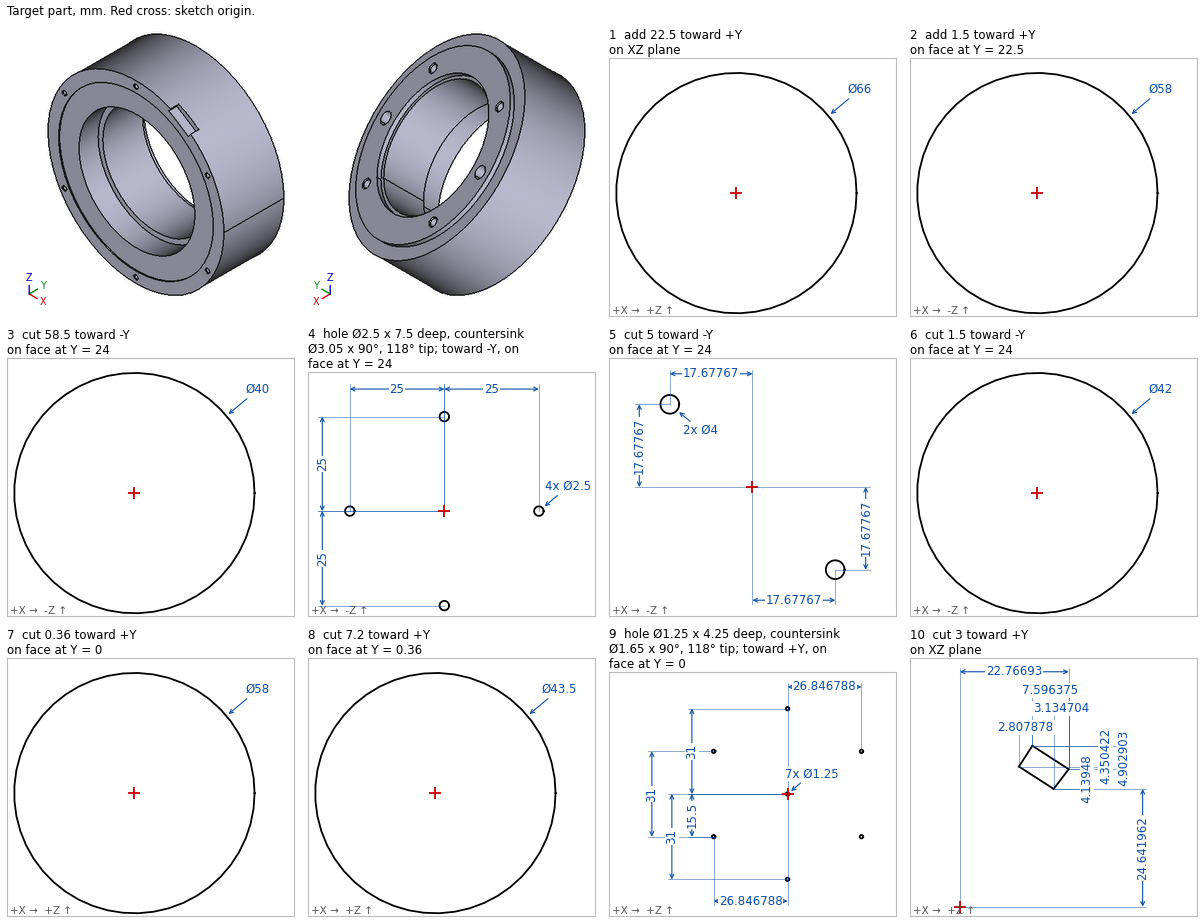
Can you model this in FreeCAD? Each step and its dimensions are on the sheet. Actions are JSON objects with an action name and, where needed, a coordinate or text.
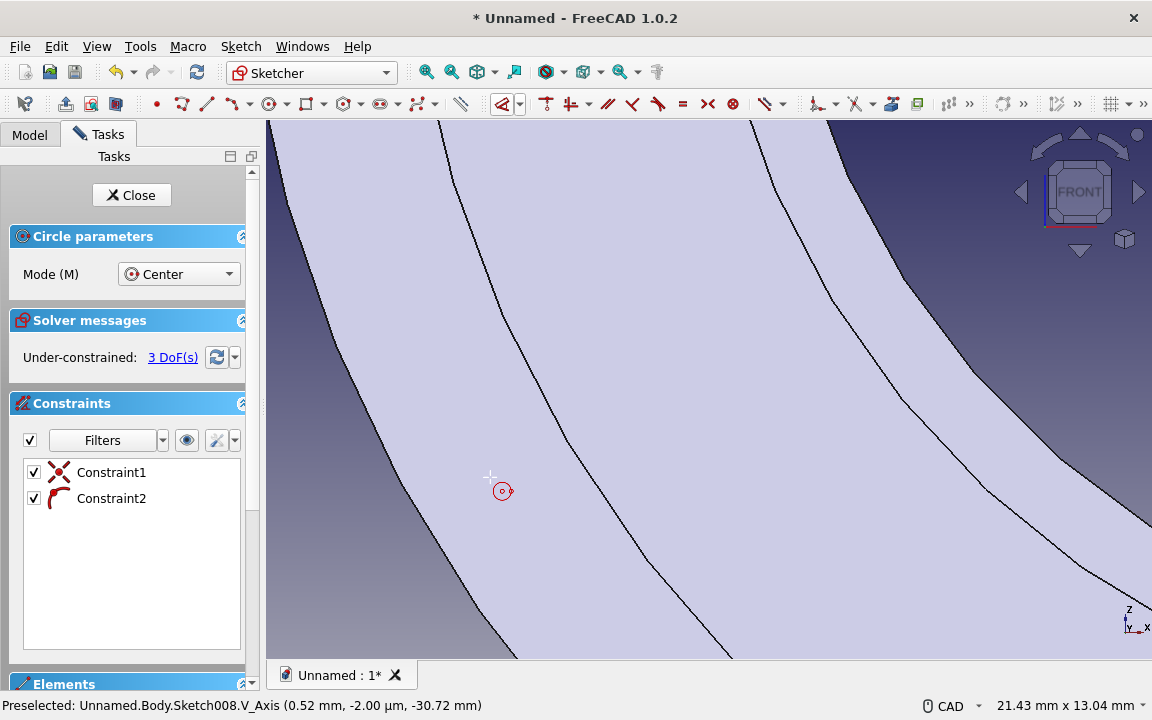
{"action": "scroll", "coordinate": [490, 477], "scroll_direction": "down", "scroll_amount": 10}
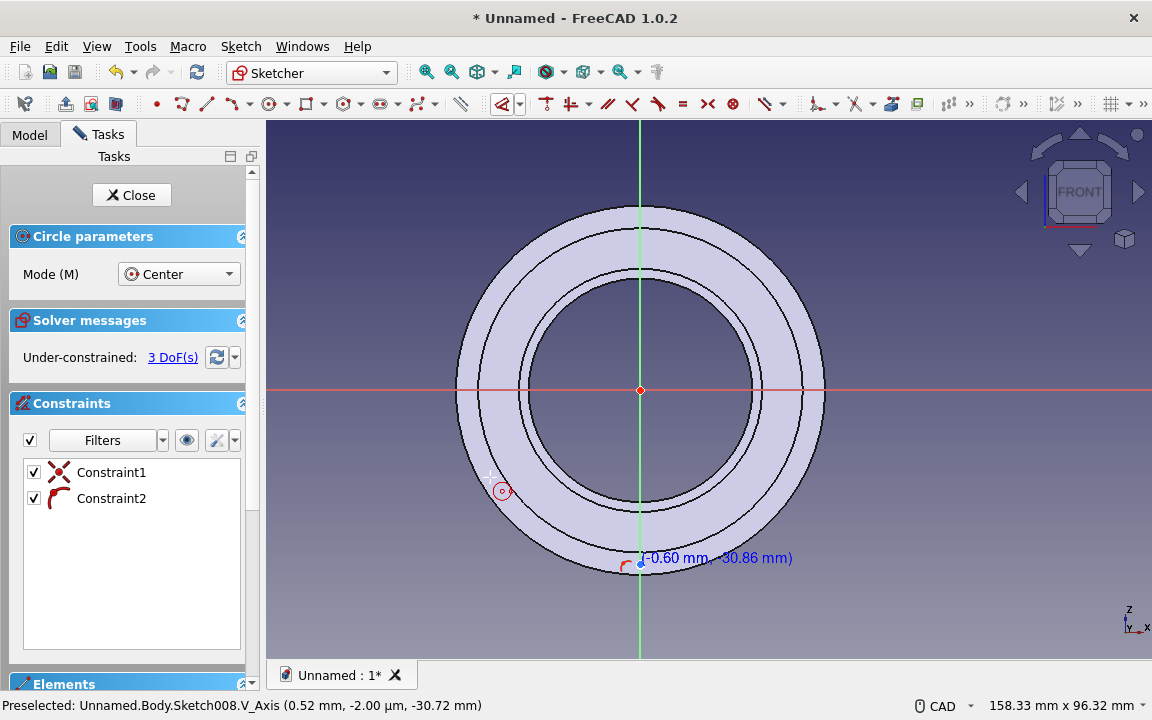
{"action": "left_click", "coordinate": [490, 477]}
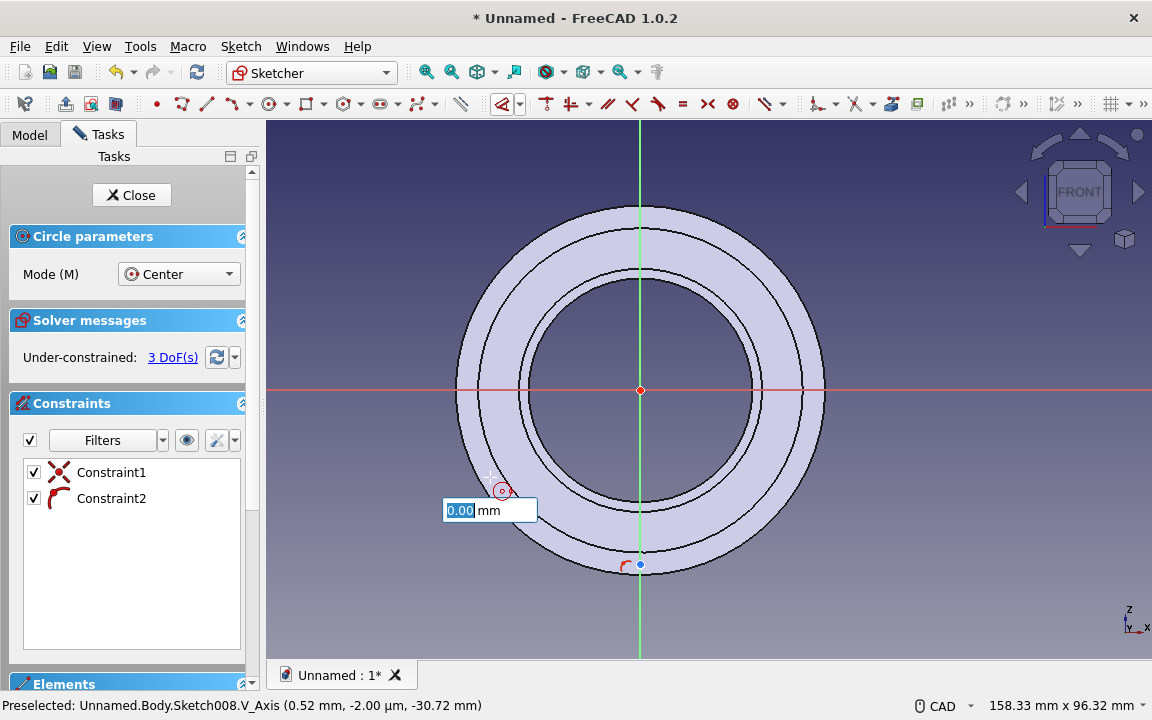
{"action": "scroll", "coordinate": [493, 475], "scroll_direction": "up", "scroll_amount": 8}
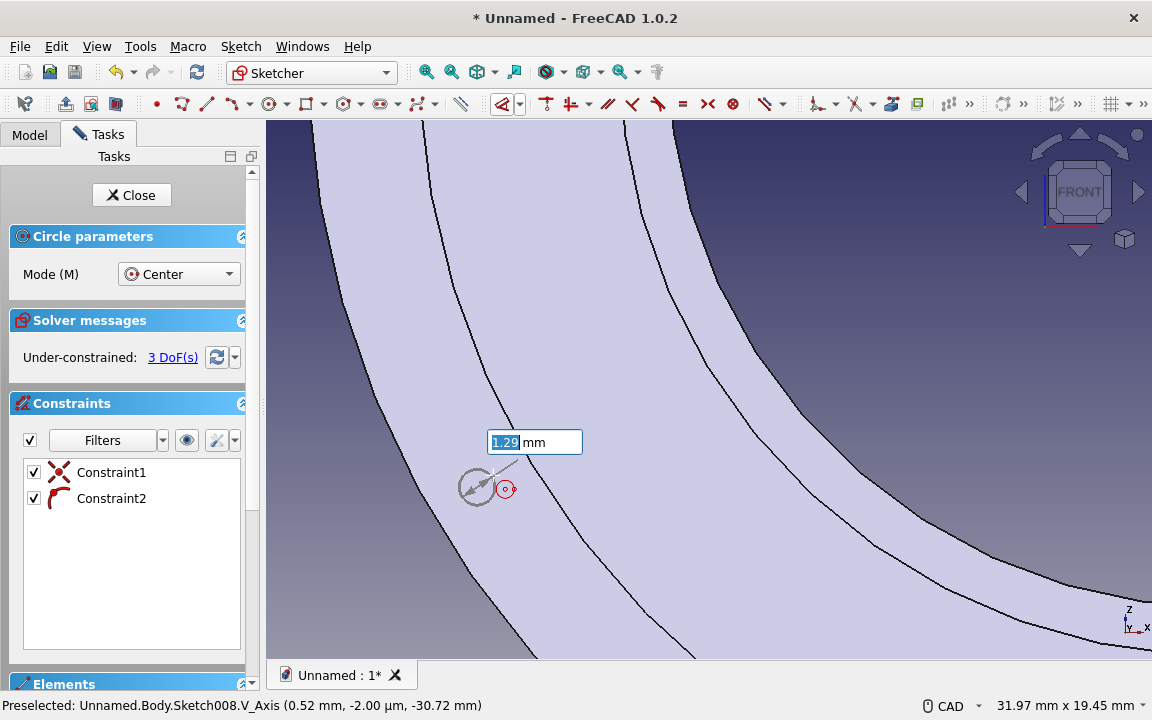
{"action": "left_click", "coordinate": [491, 471]}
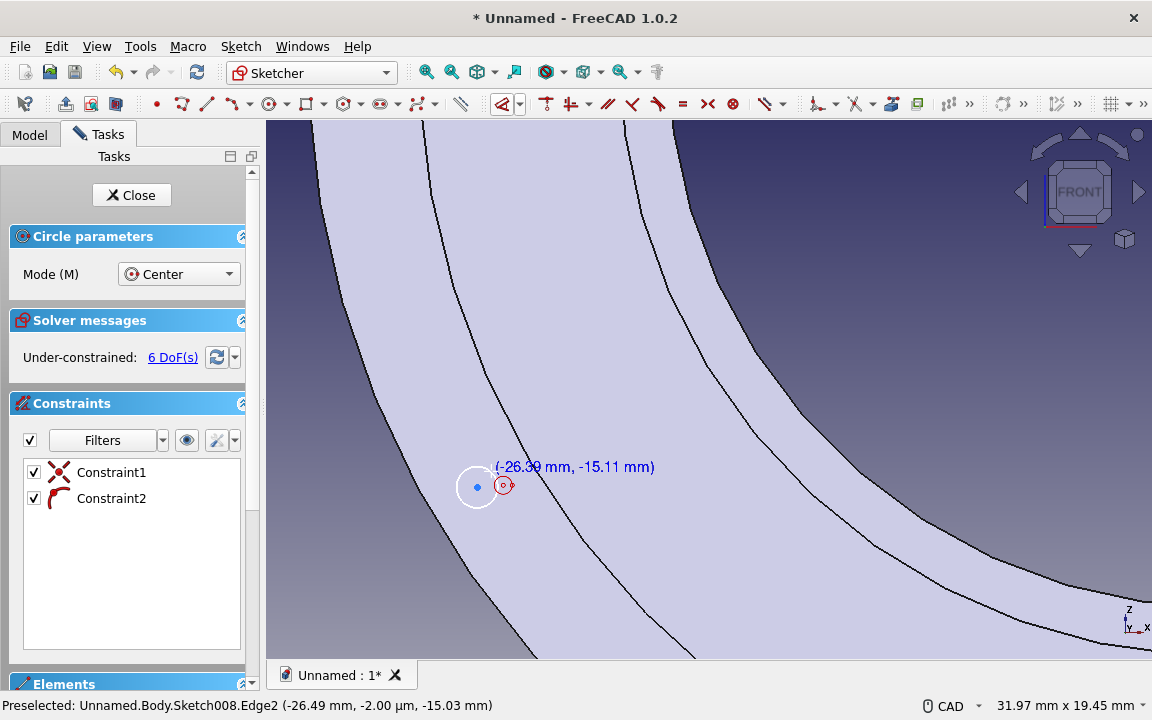
{"action": "scroll", "coordinate": [493, 475], "scroll_direction": "down", "scroll_amount": 8}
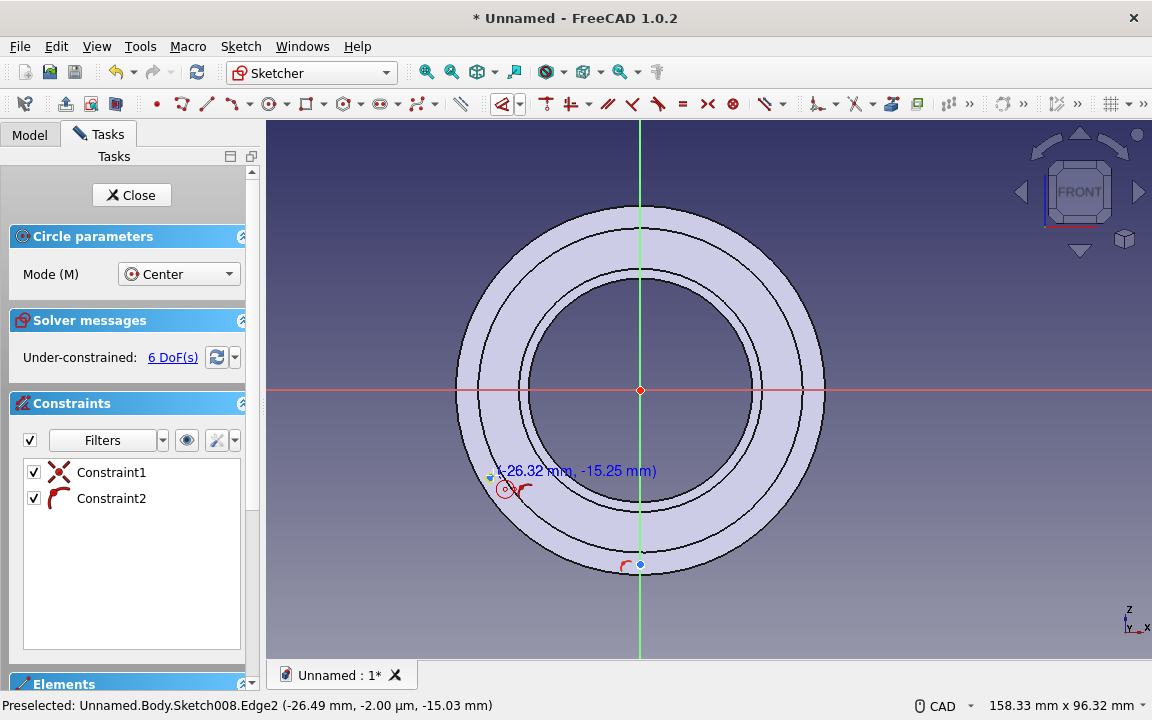
{"action": "scroll", "coordinate": [490, 304], "scroll_direction": "up", "scroll_amount": 10}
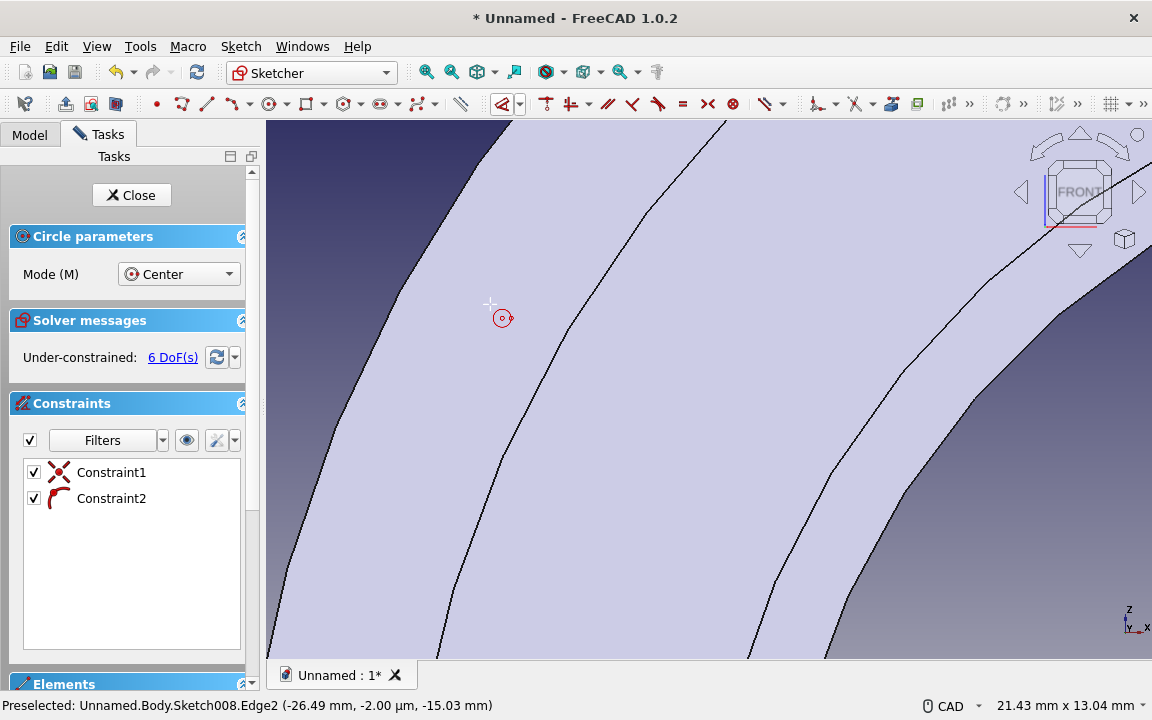
{"action": "scroll", "coordinate": [490, 303], "scroll_direction": "down", "scroll_amount": 10}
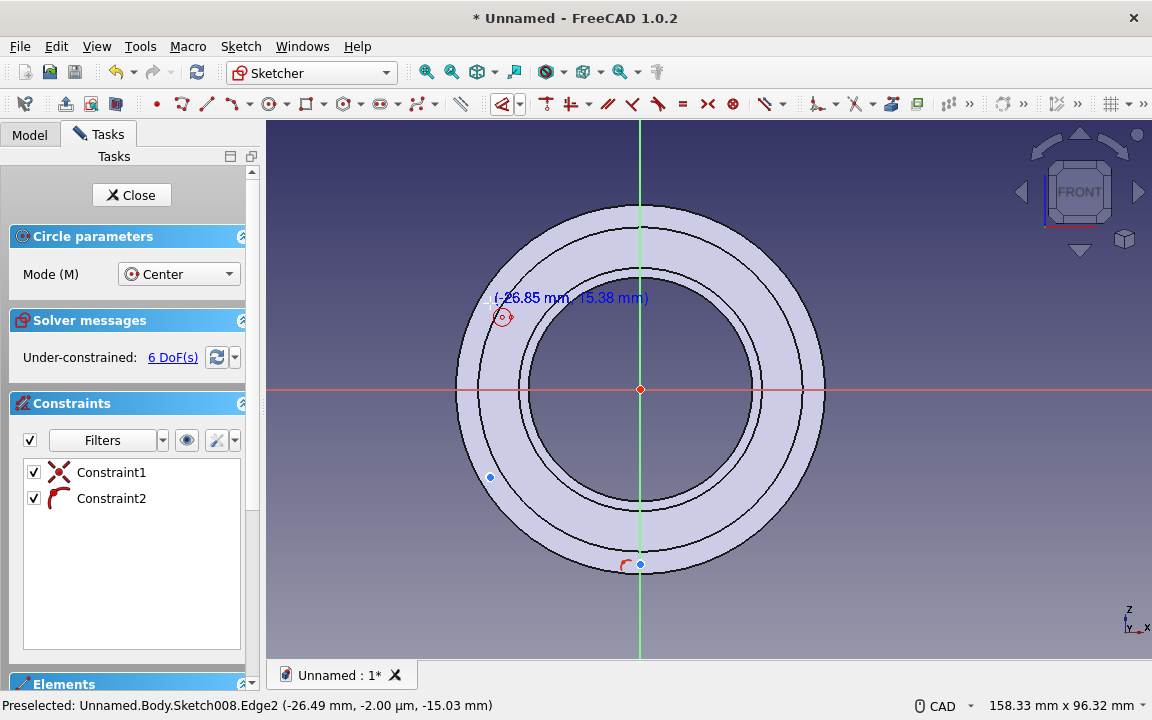
{"action": "left_click", "coordinate": [490, 303]}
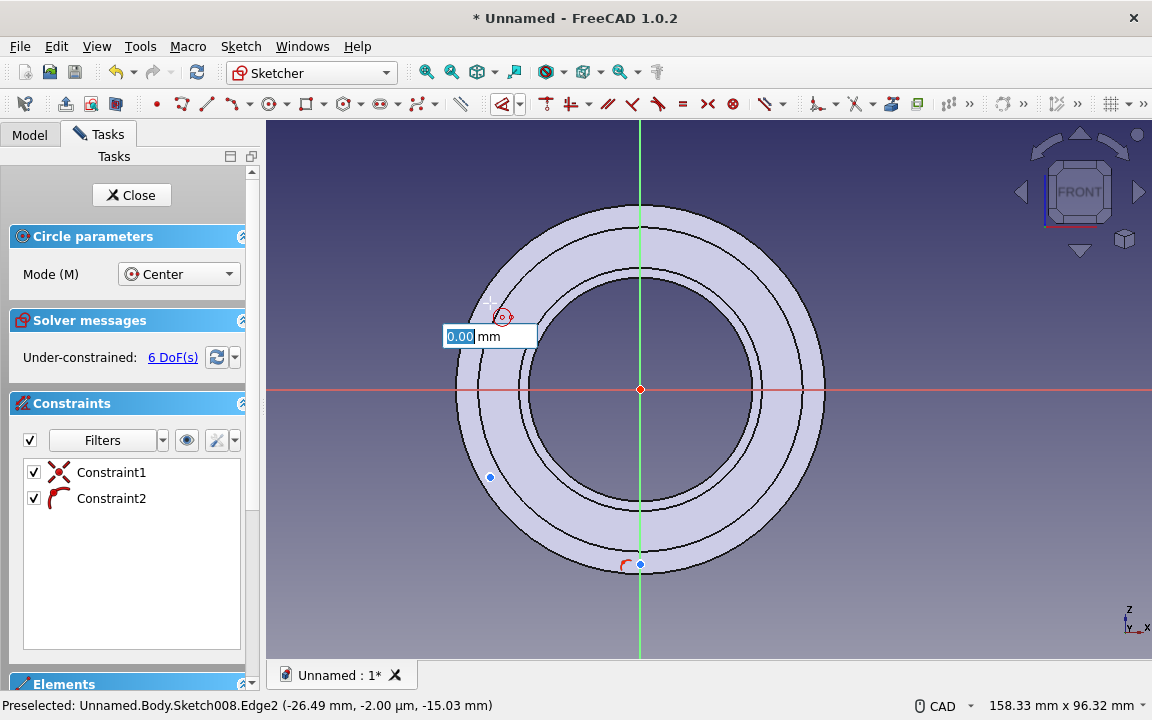
{"action": "scroll", "coordinate": [493, 300], "scroll_direction": "up", "scroll_amount": 8}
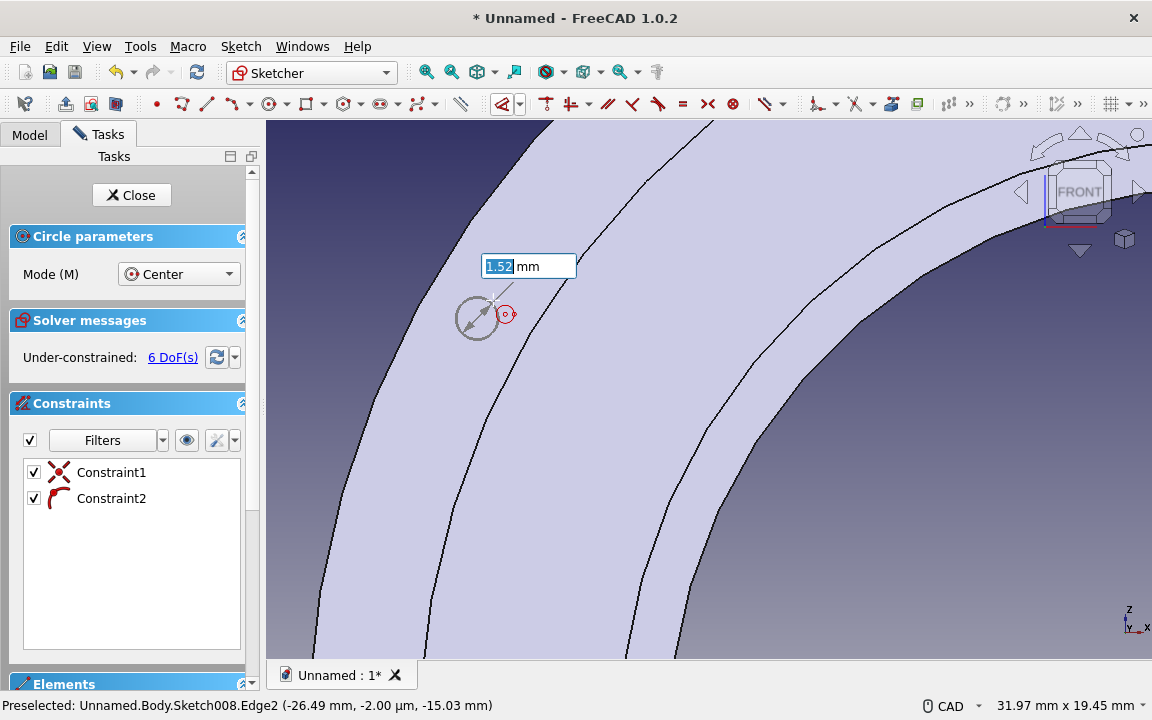
{"action": "left_click", "coordinate": [491, 300]}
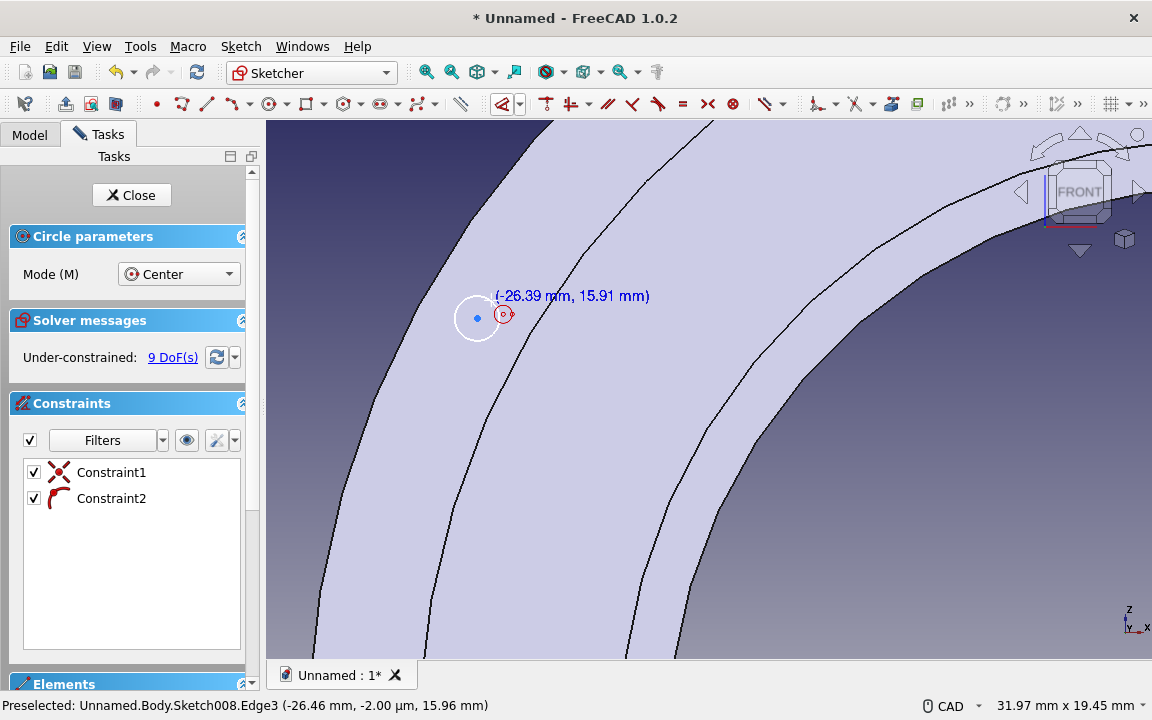
{"action": "scroll", "coordinate": [493, 300], "scroll_direction": "down", "scroll_amount": 8}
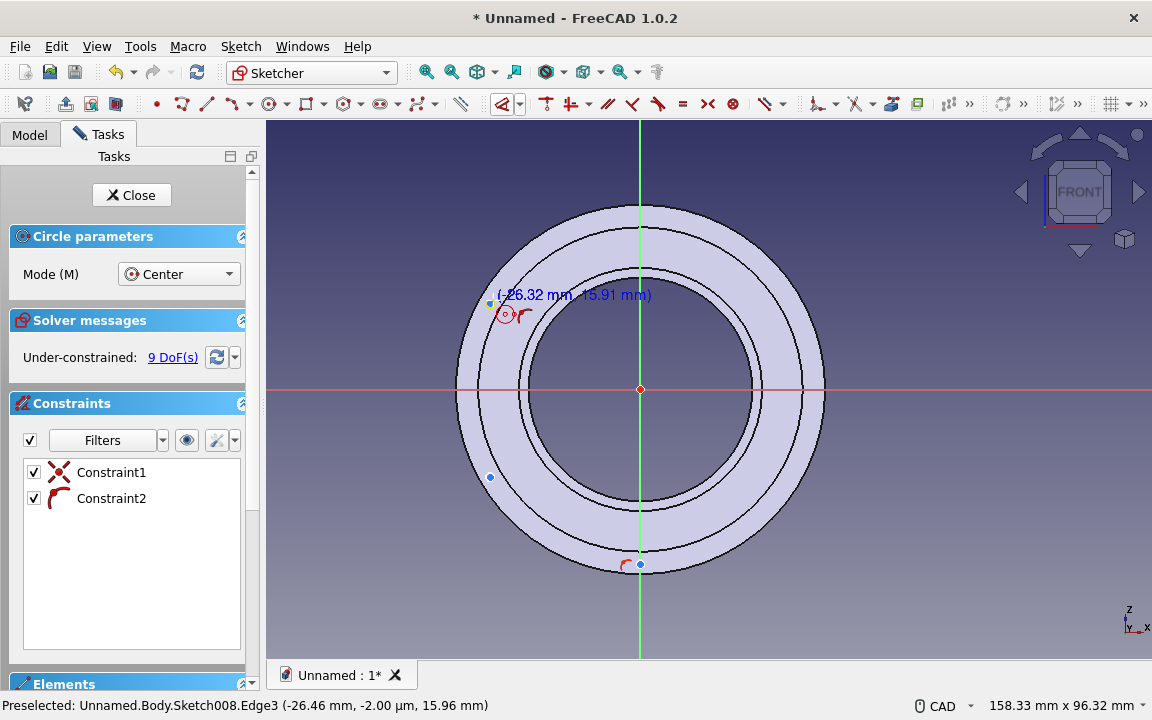
{"action": "scroll", "coordinate": [640, 216], "scroll_direction": "up", "scroll_amount": 10}